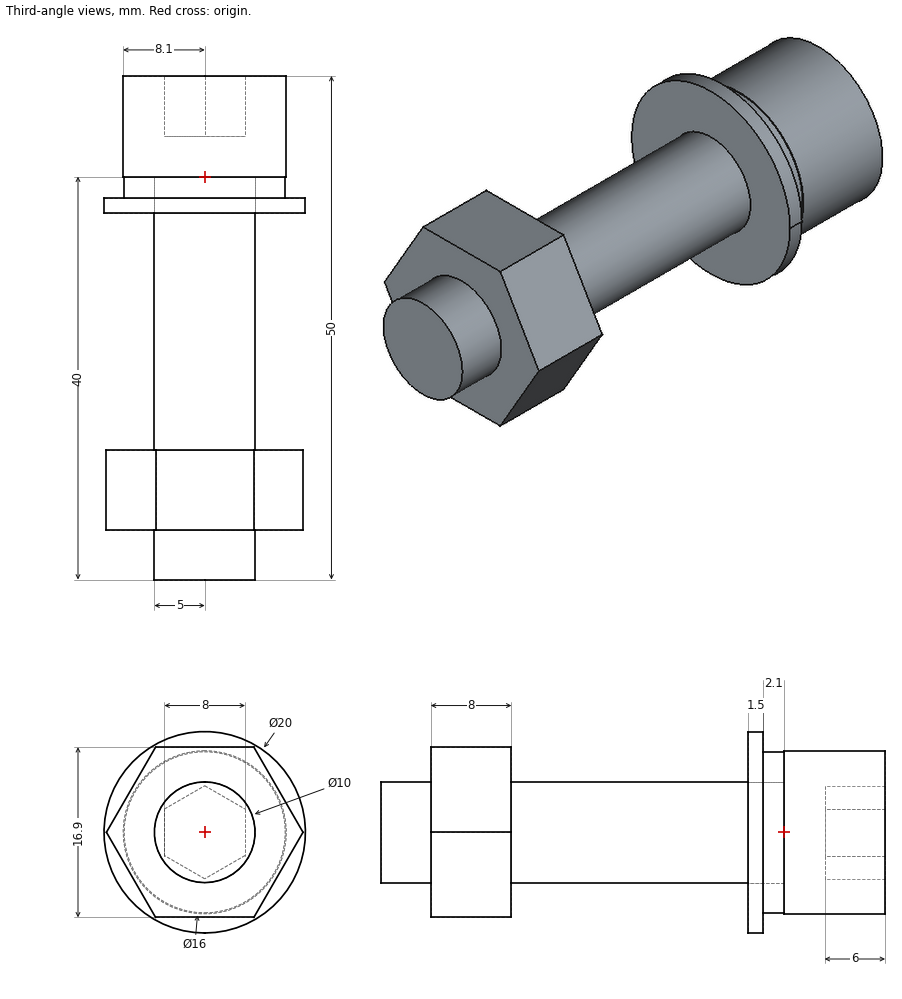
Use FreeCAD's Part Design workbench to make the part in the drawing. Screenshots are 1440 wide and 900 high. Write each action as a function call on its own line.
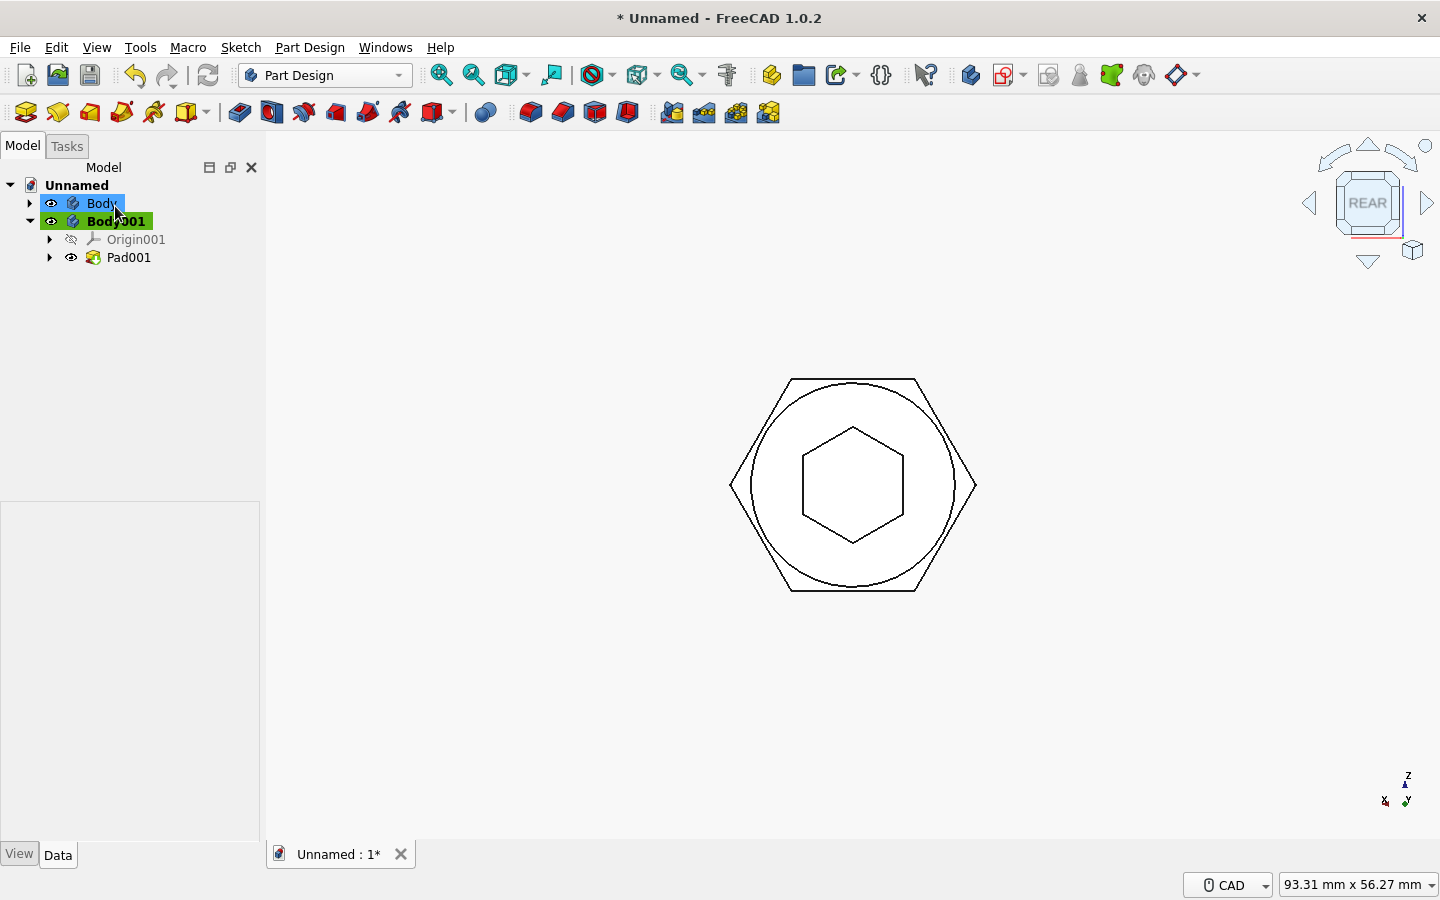
click(442, 76)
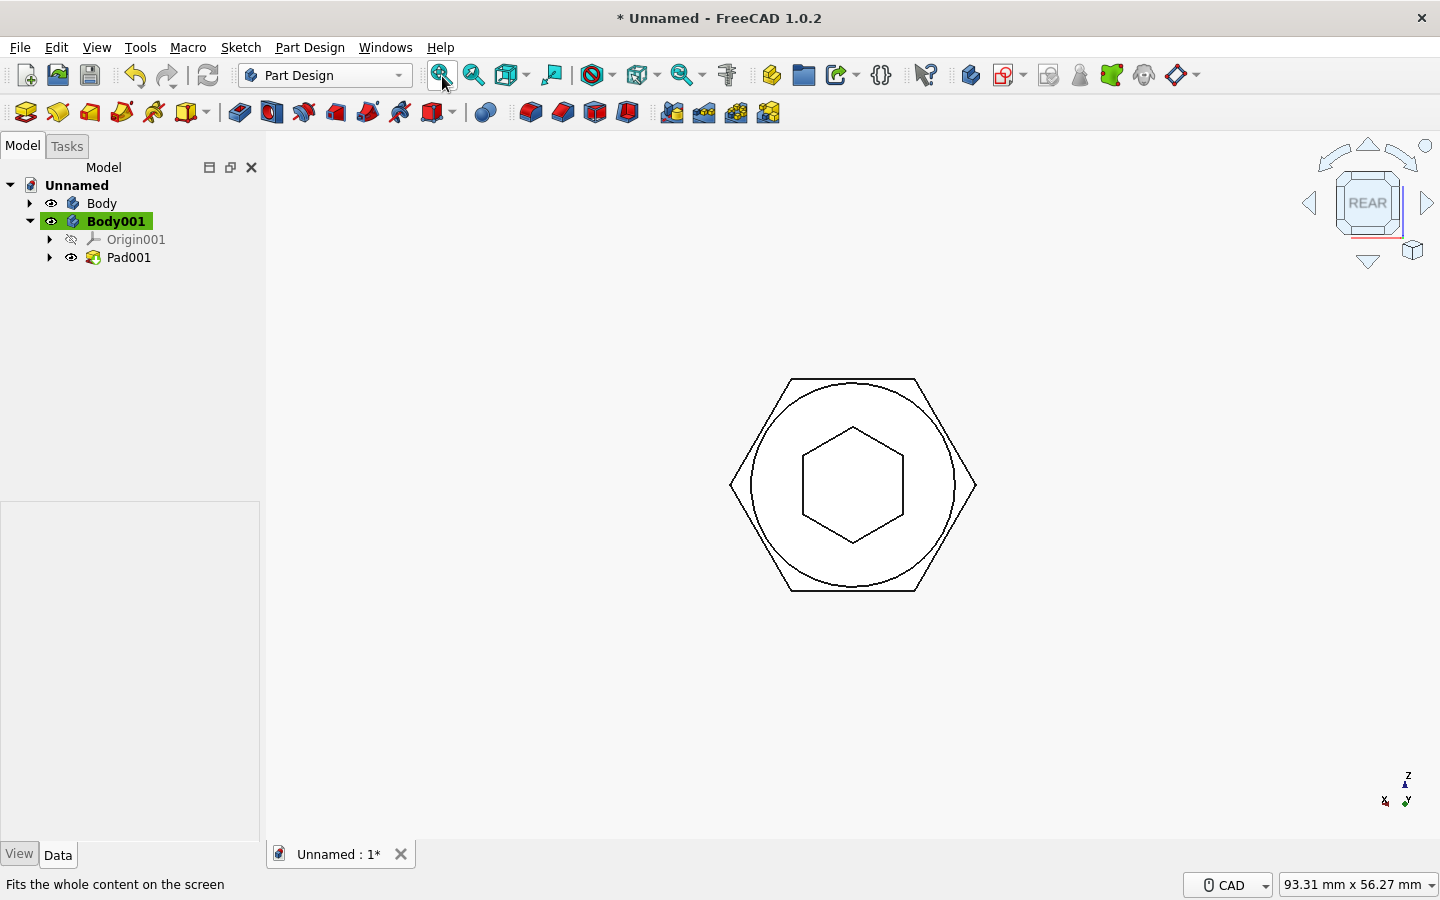
click(972, 76)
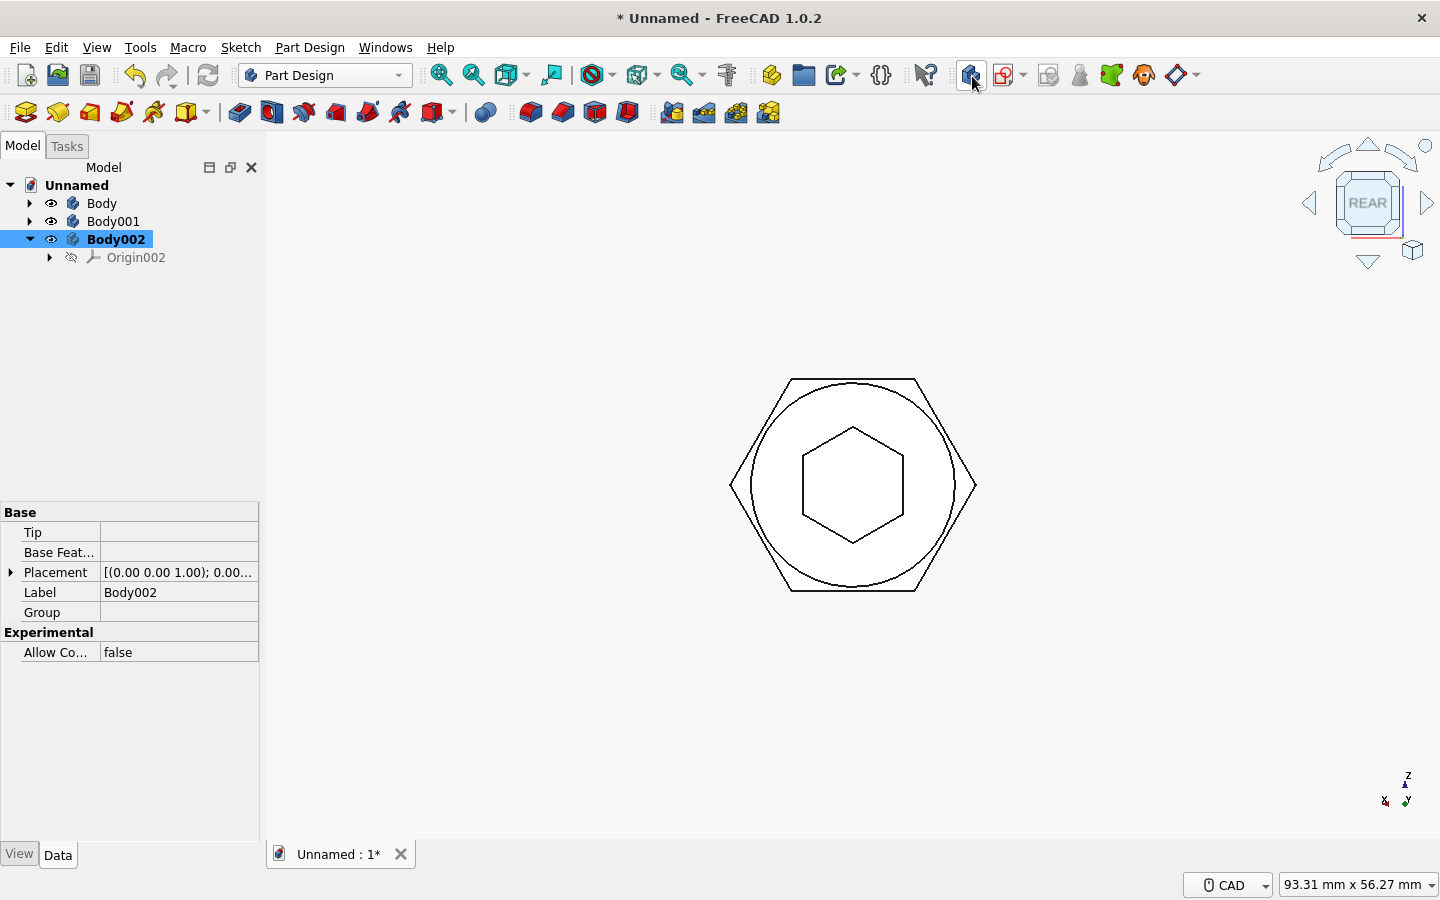
click(50, 257)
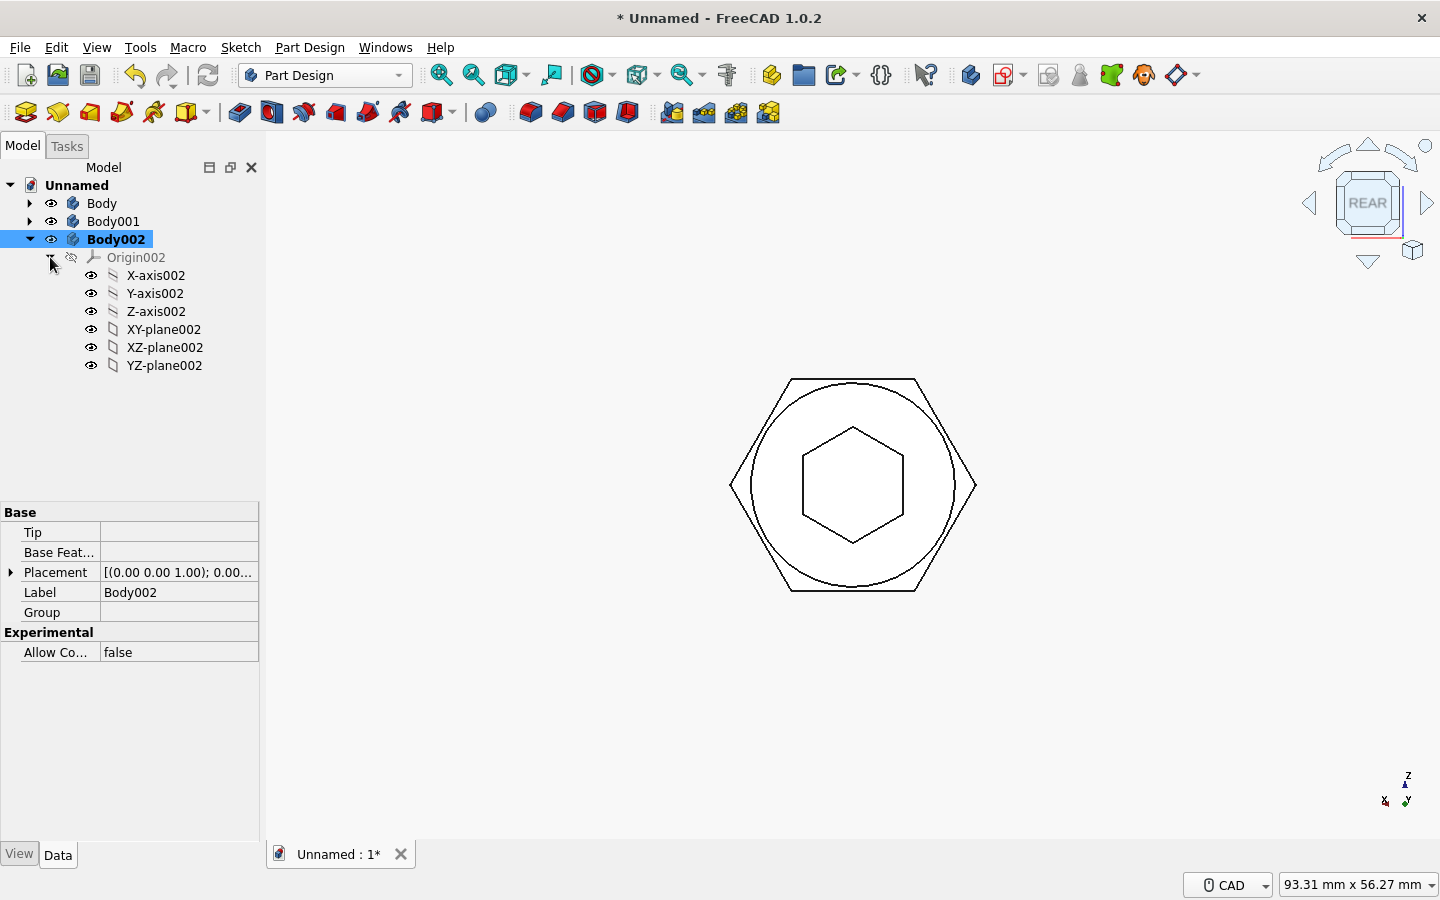
click(136, 347)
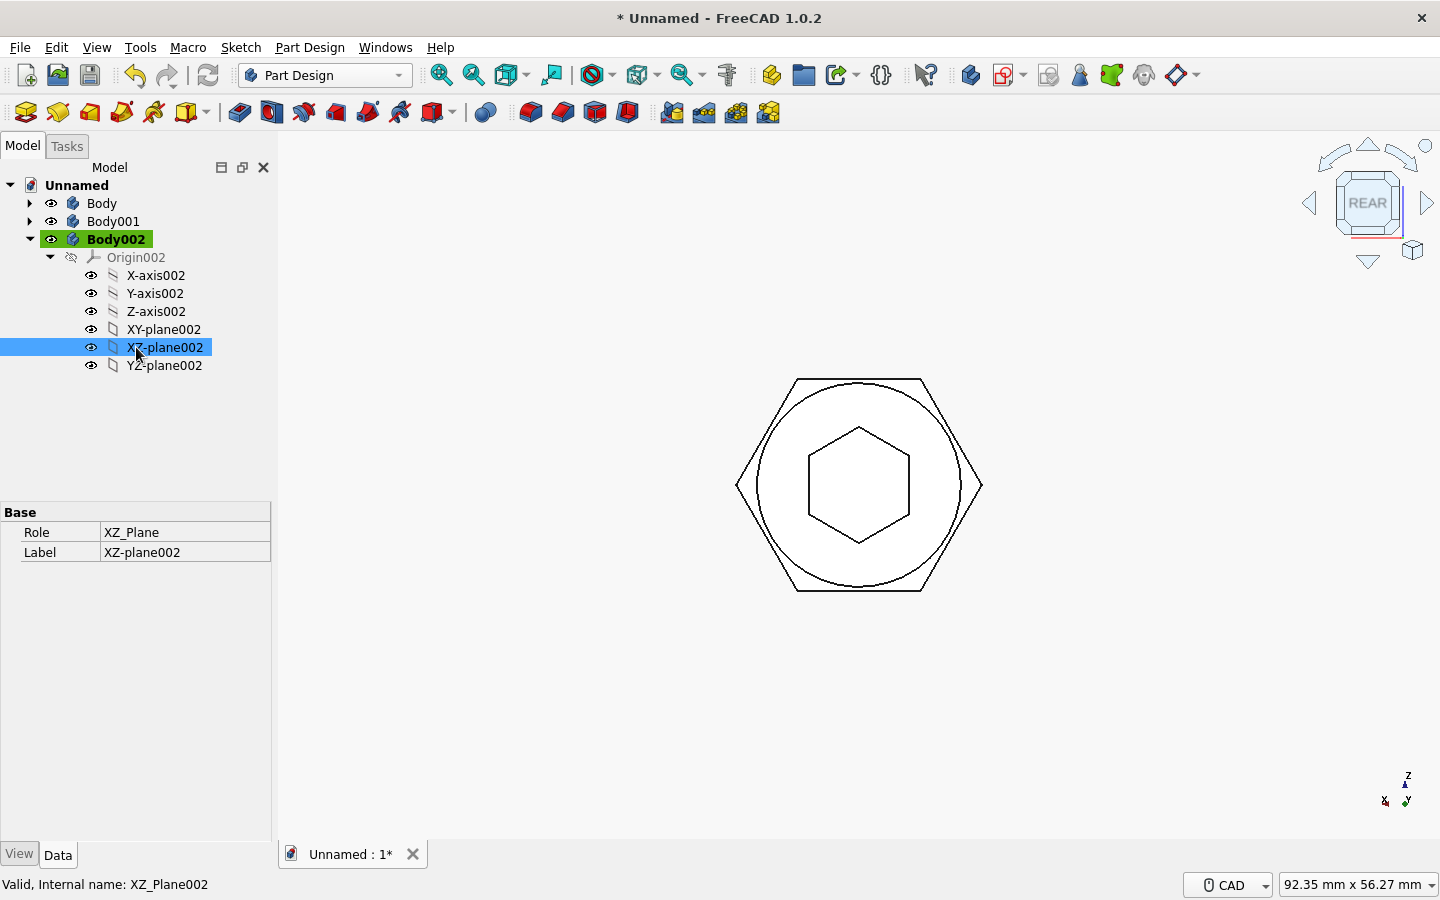
click(1176, 76)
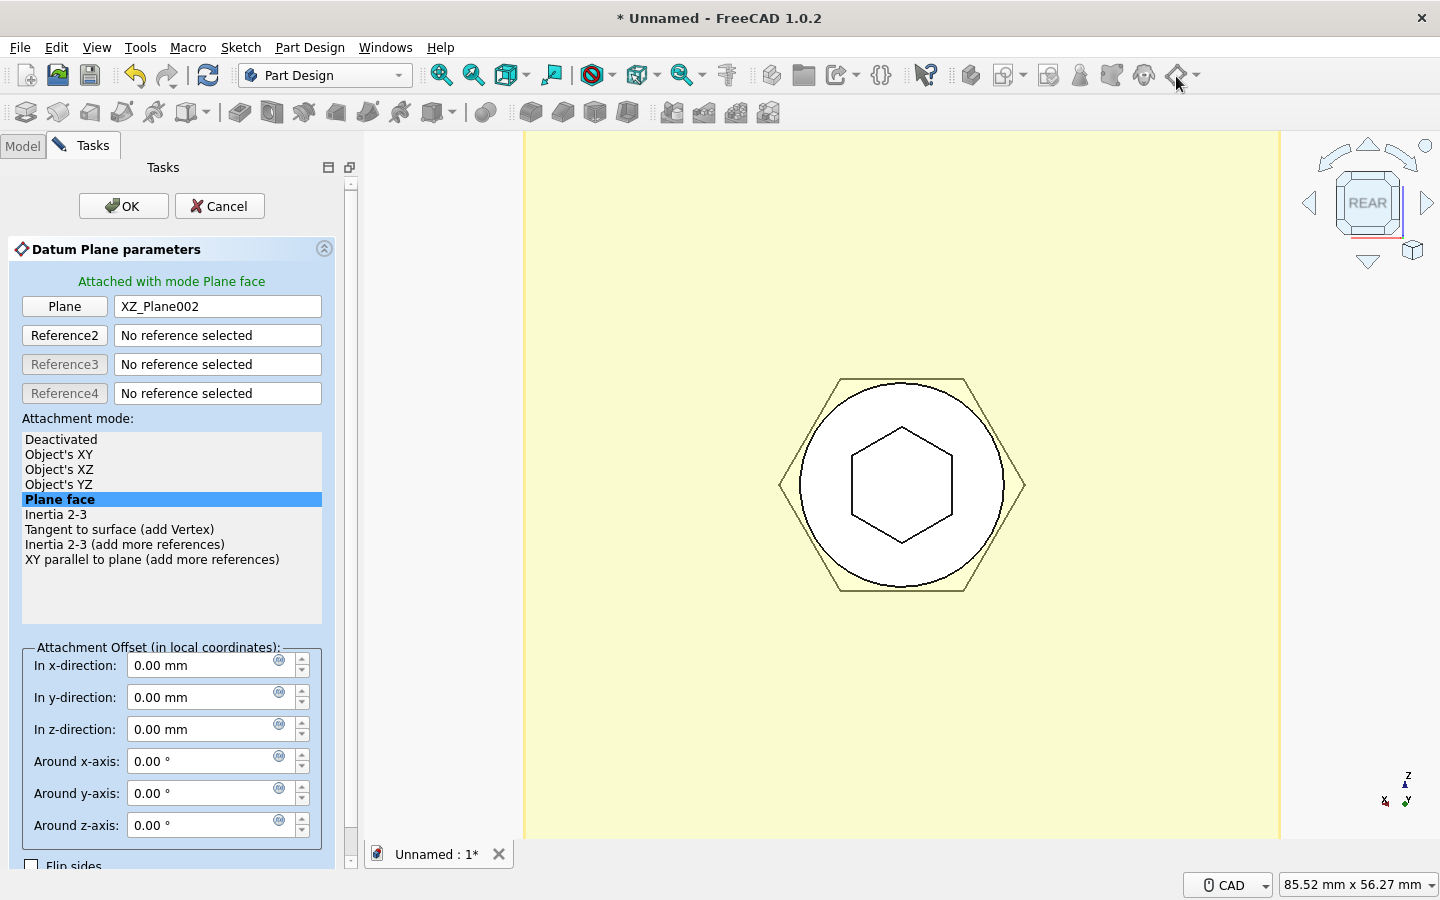
triple_click(210, 729)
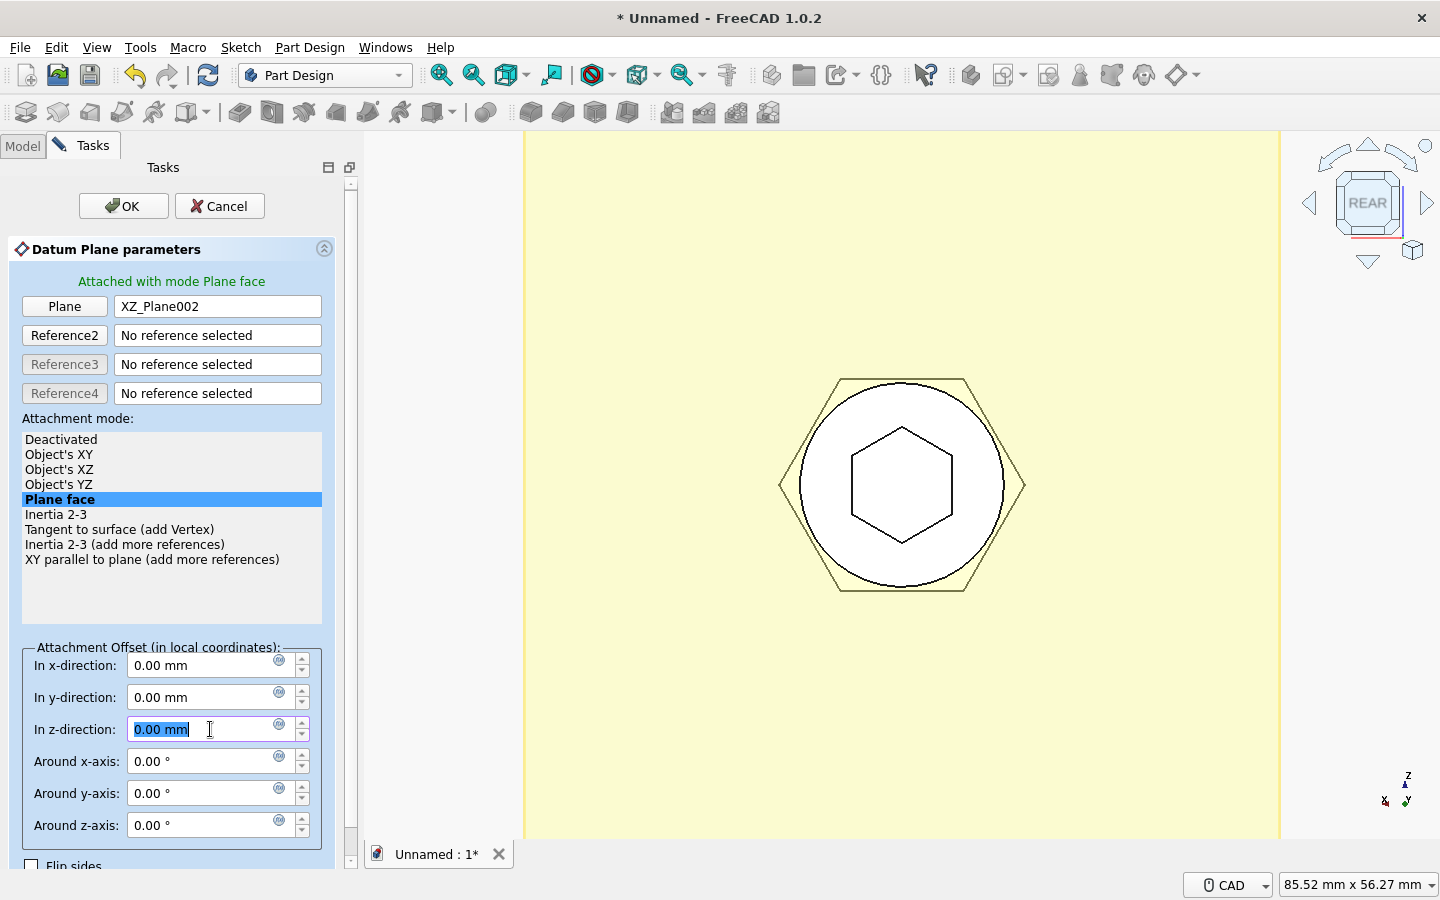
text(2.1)
key(Tab)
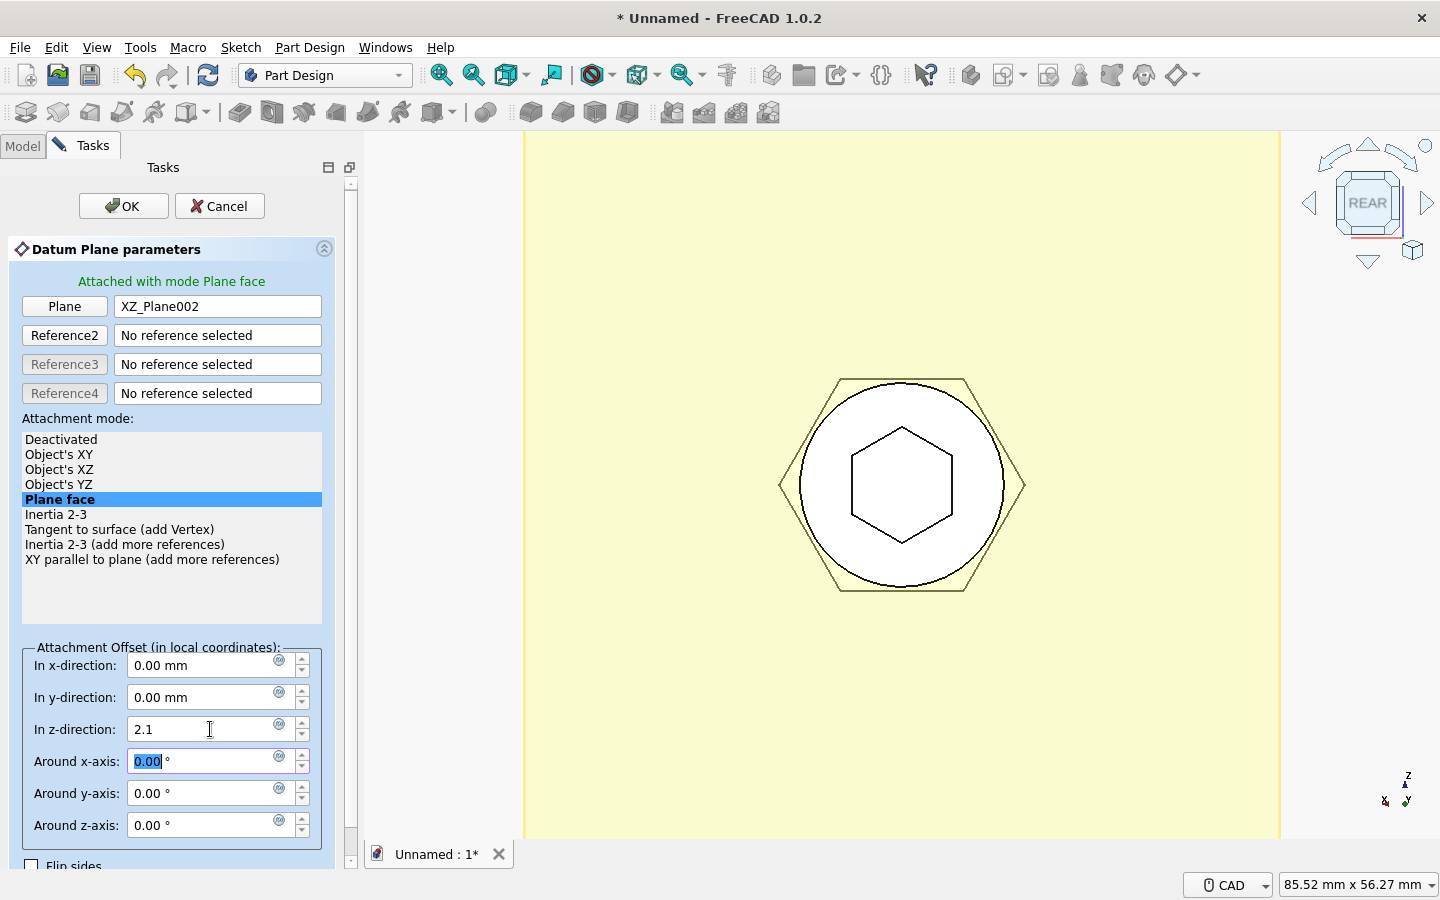
click(124, 206)